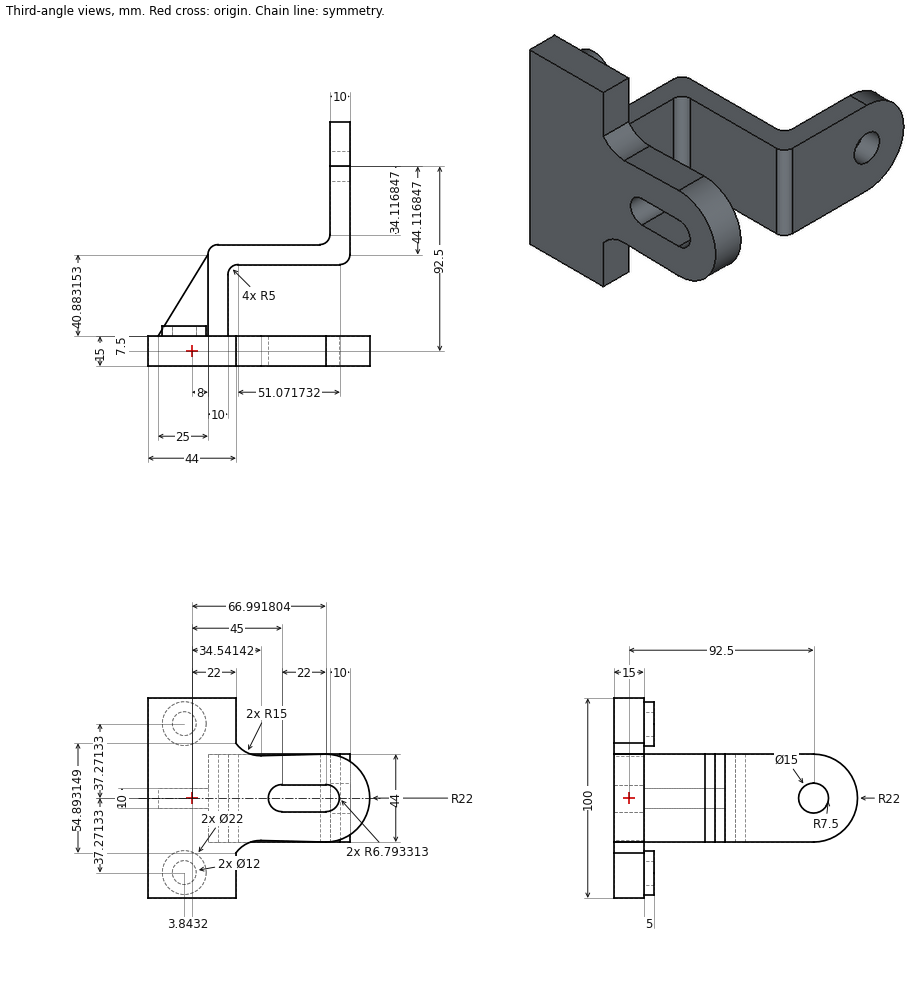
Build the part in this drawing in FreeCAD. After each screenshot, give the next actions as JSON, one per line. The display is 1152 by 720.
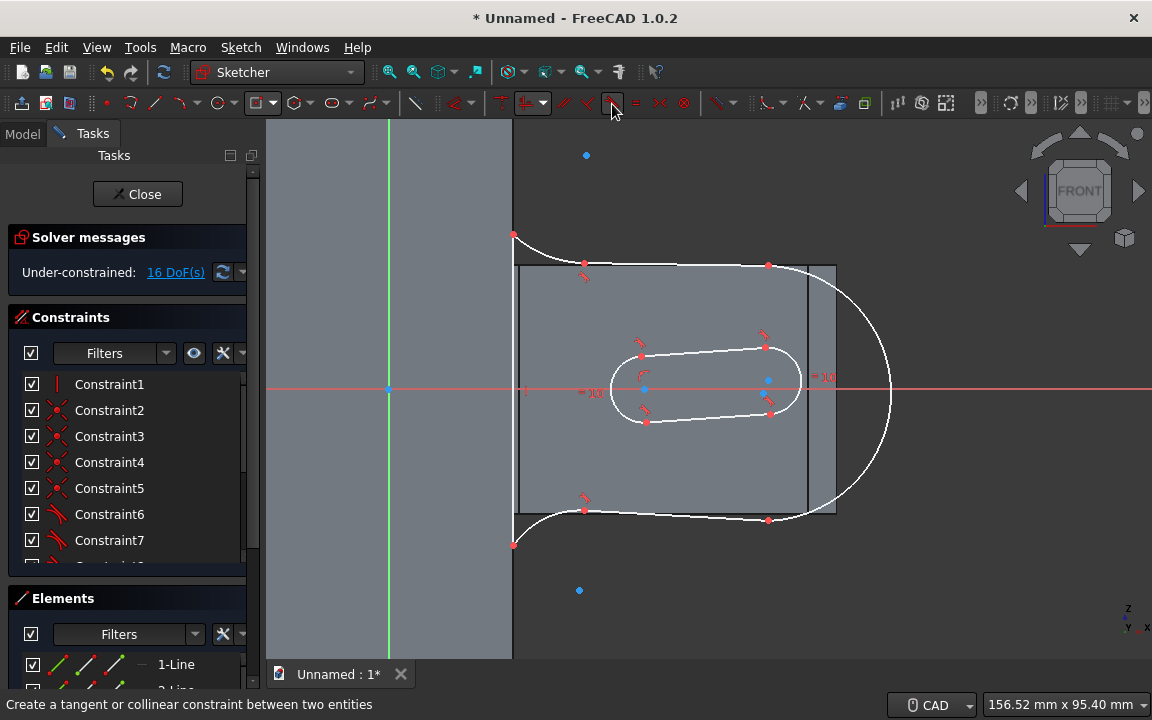
{"action": "left_click", "coordinate": [679, 354]}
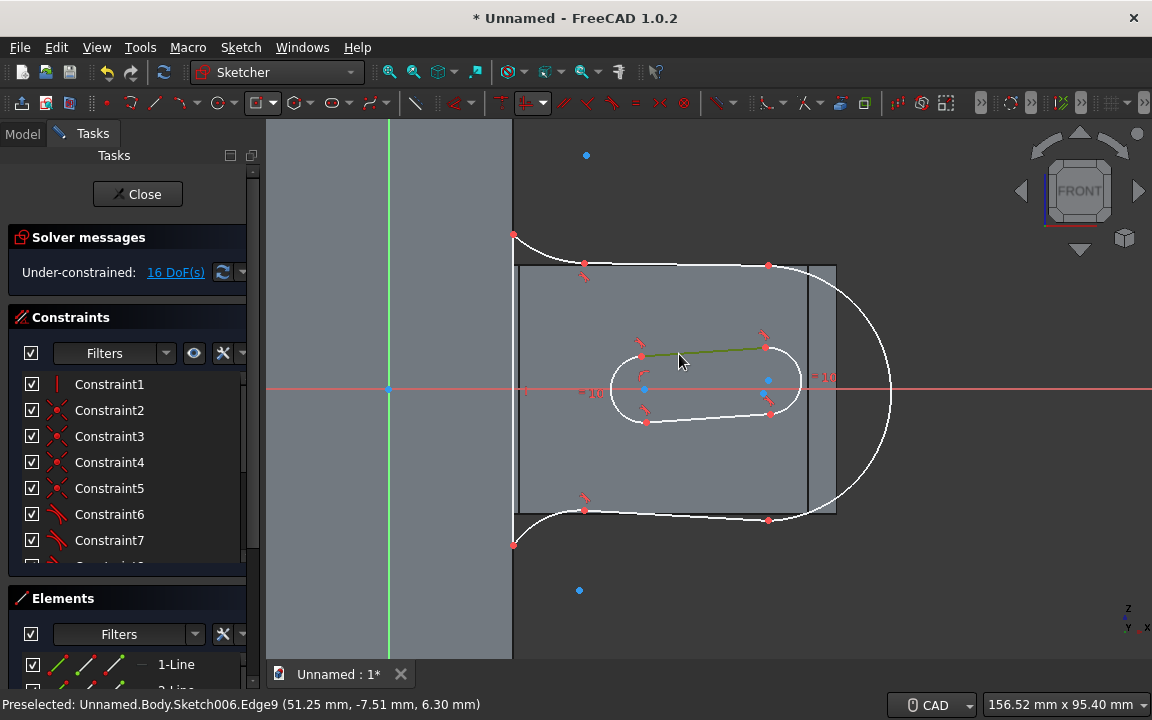
{"action": "key", "text": "h"}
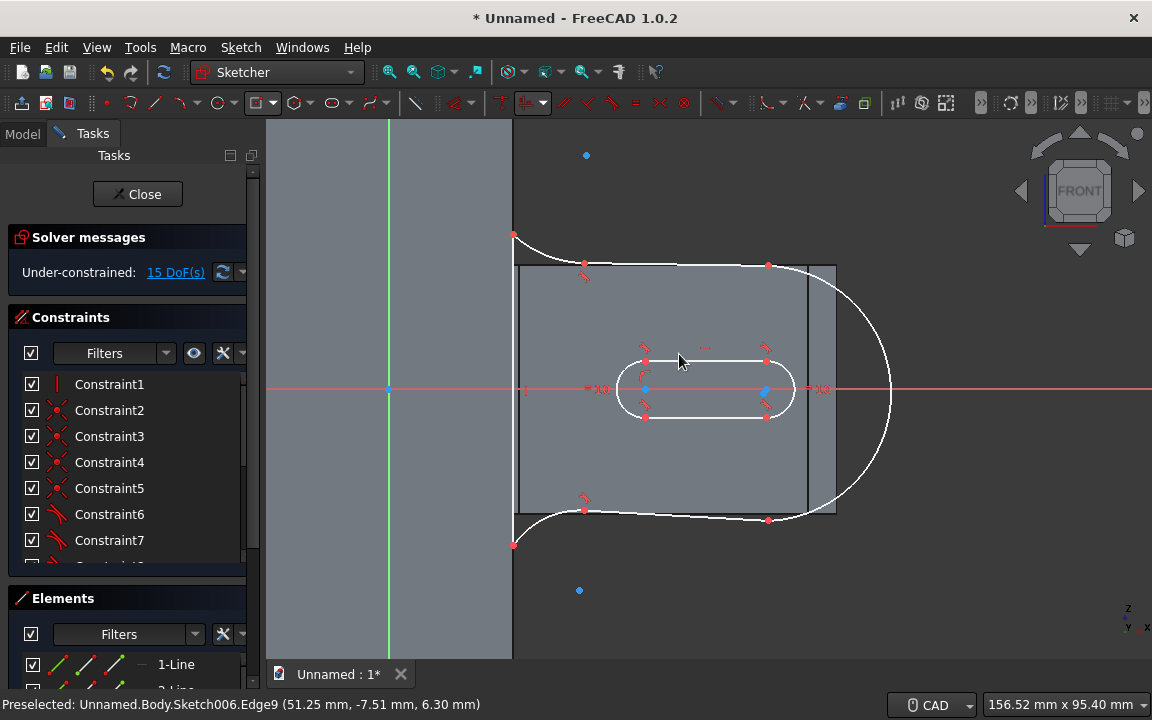
{"action": "left_click", "coordinate": [868, 467]}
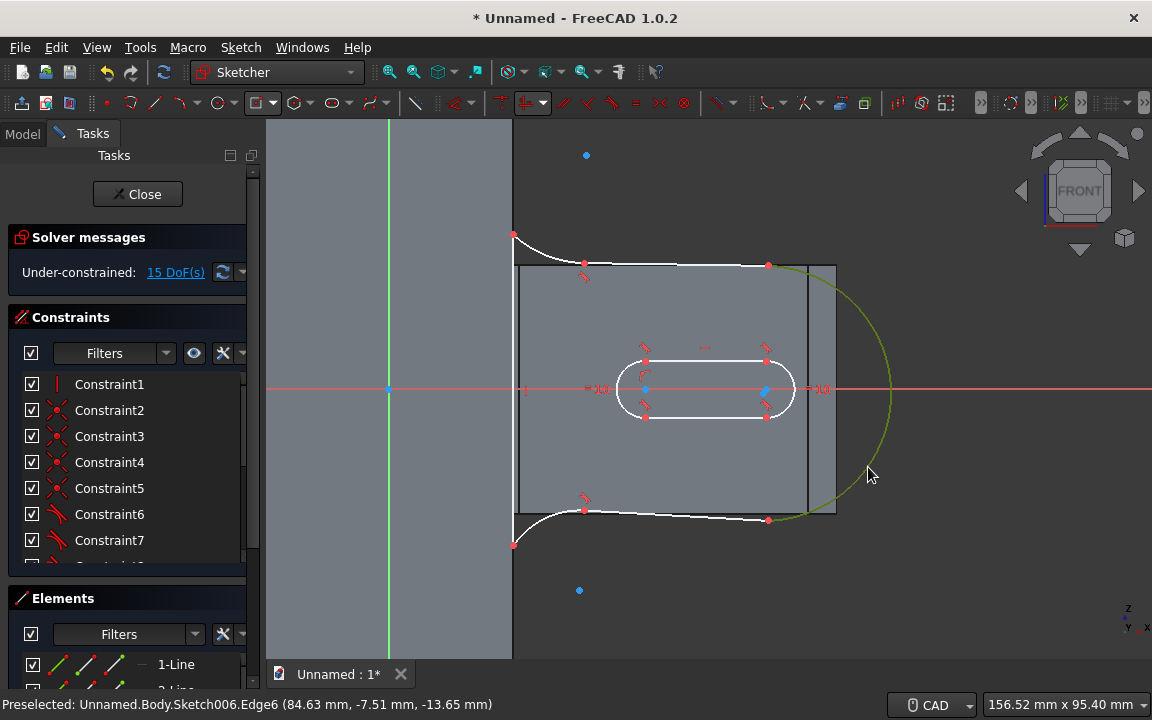
{"action": "left_click", "coordinate": [789, 406]}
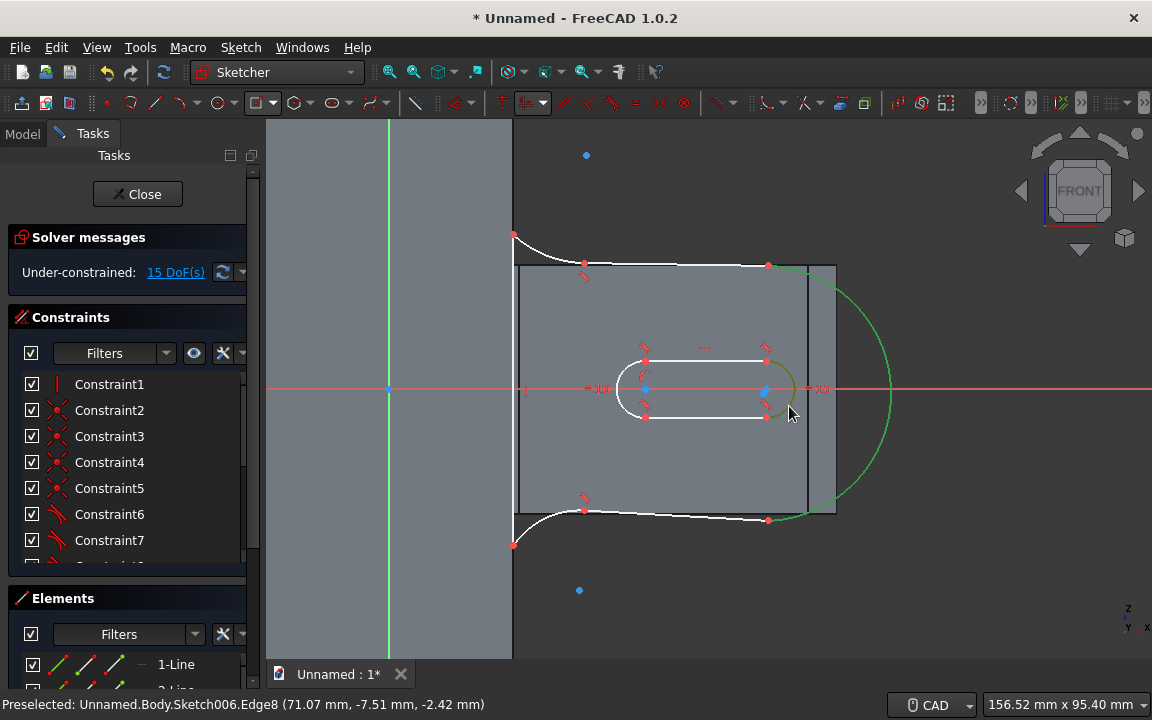
{"action": "left_click", "coordinate": [502, 104]}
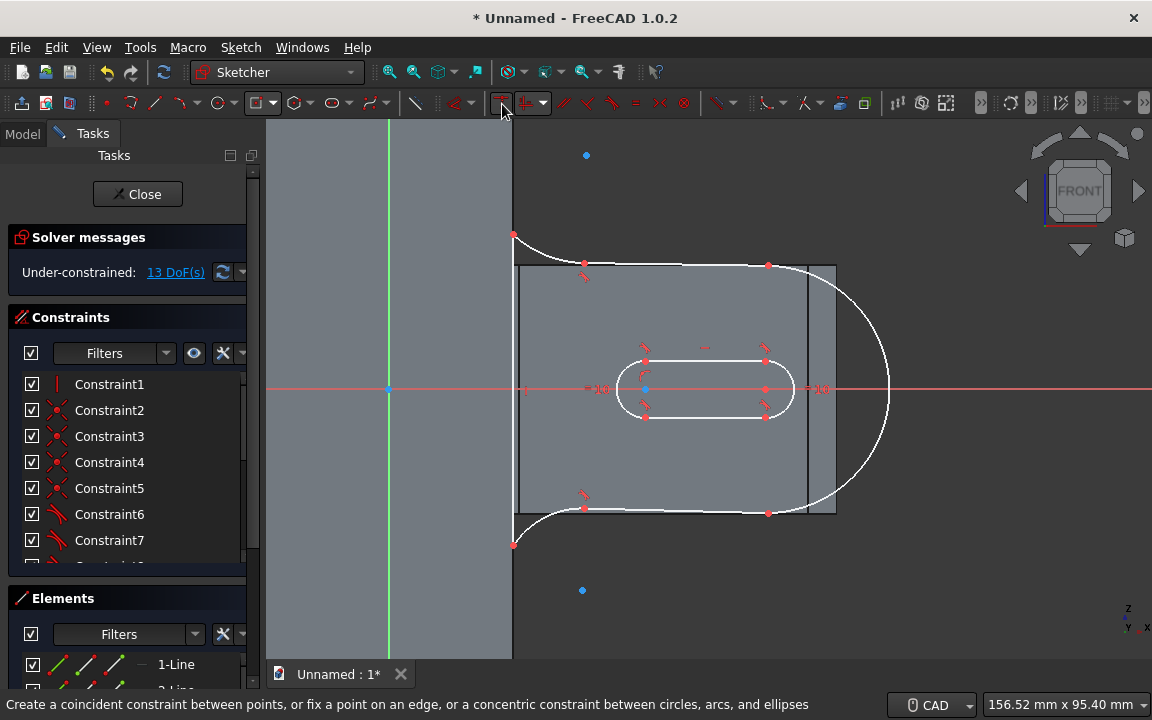
{"action": "left_click", "coordinate": [532, 249]}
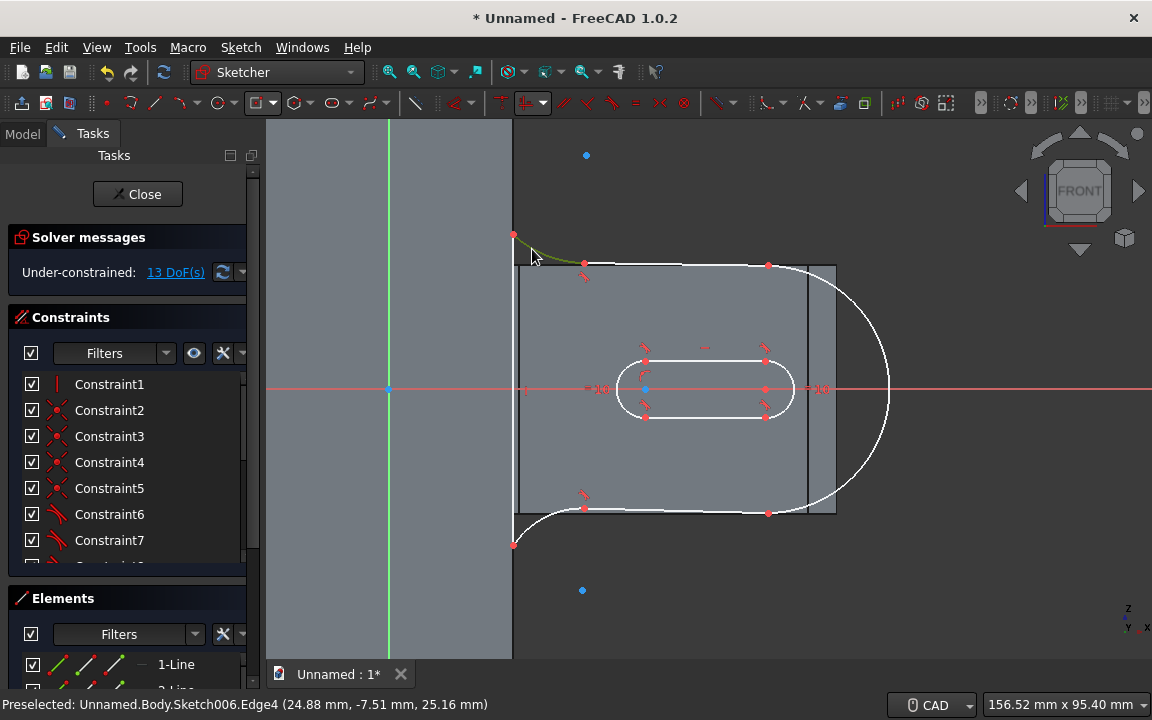
{"action": "left_click", "coordinate": [560, 512]}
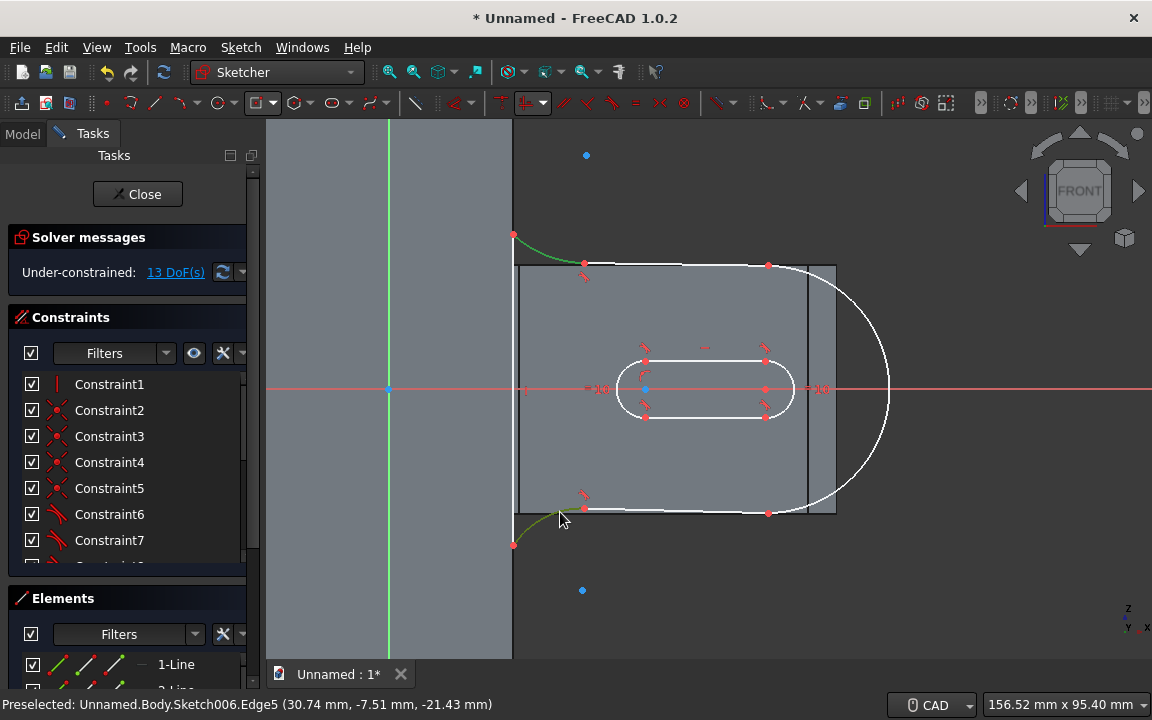
{"action": "left_click", "coordinate": [636, 104]}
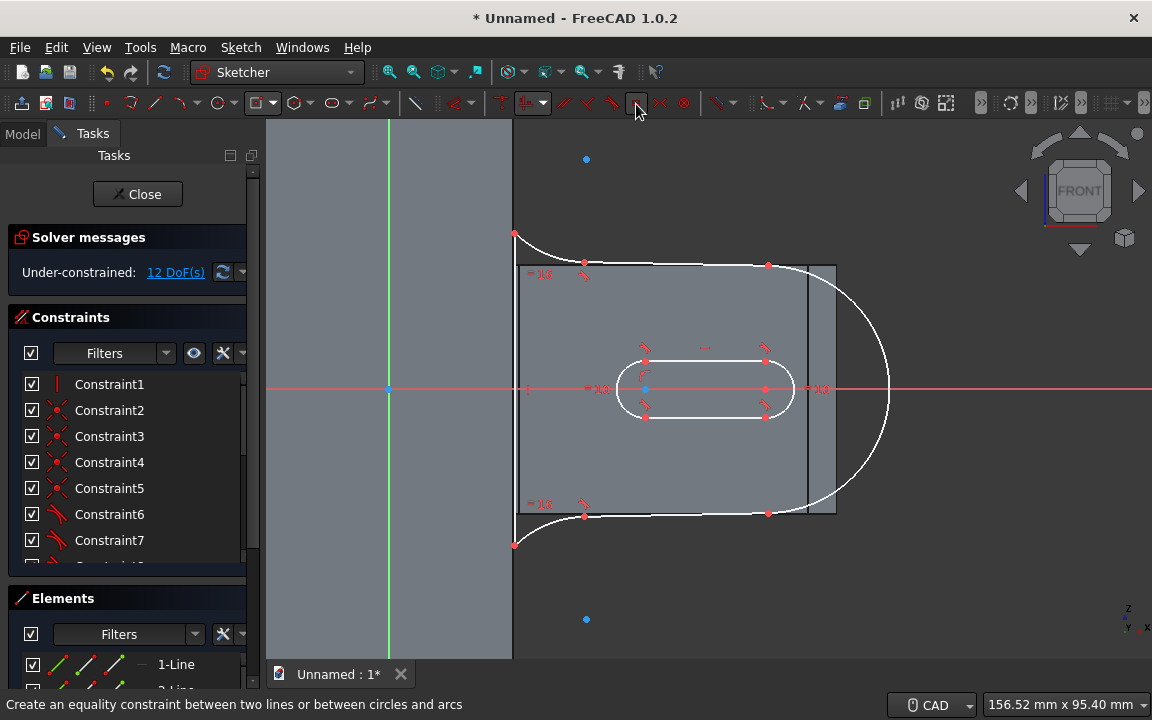
{"action": "left_click", "coordinate": [587, 160]}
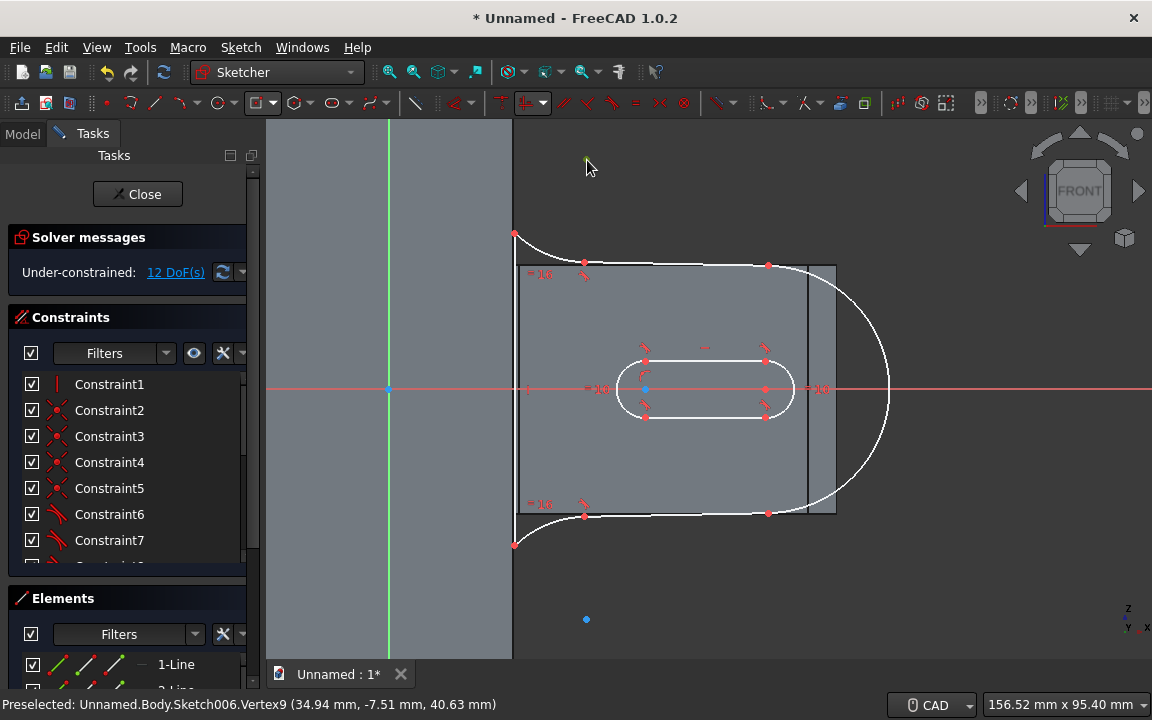
{"action": "left_click", "coordinate": [586, 619]}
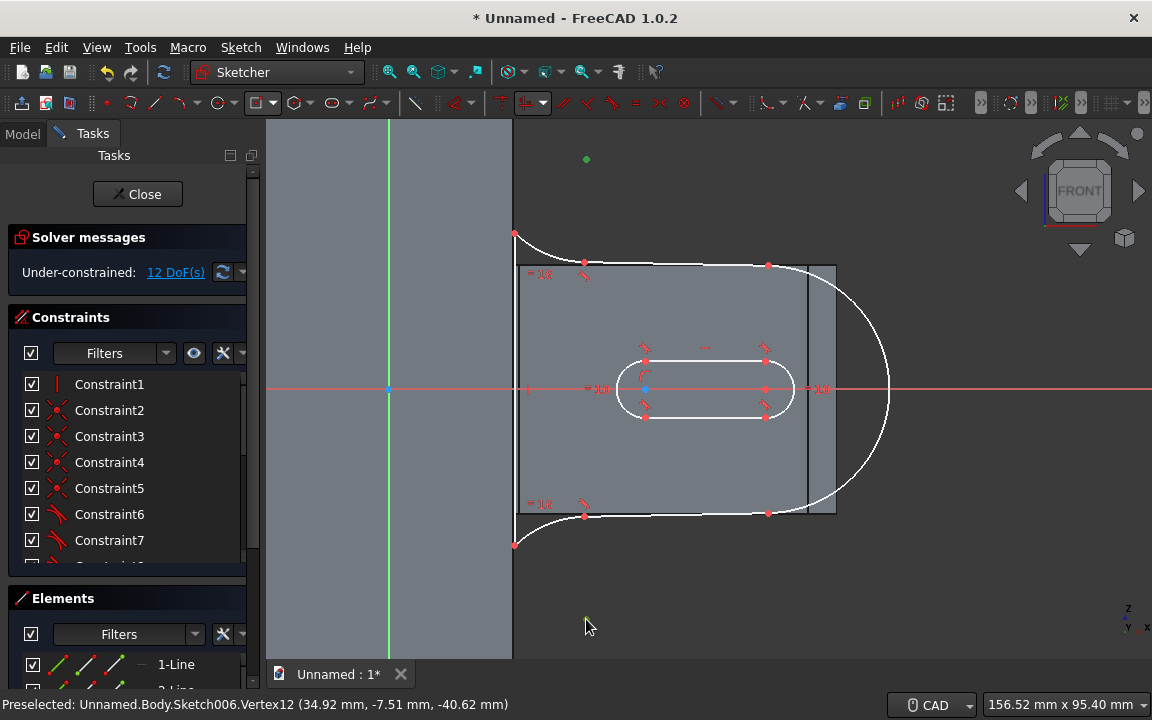
{"action": "left_click", "coordinate": [344, 389]}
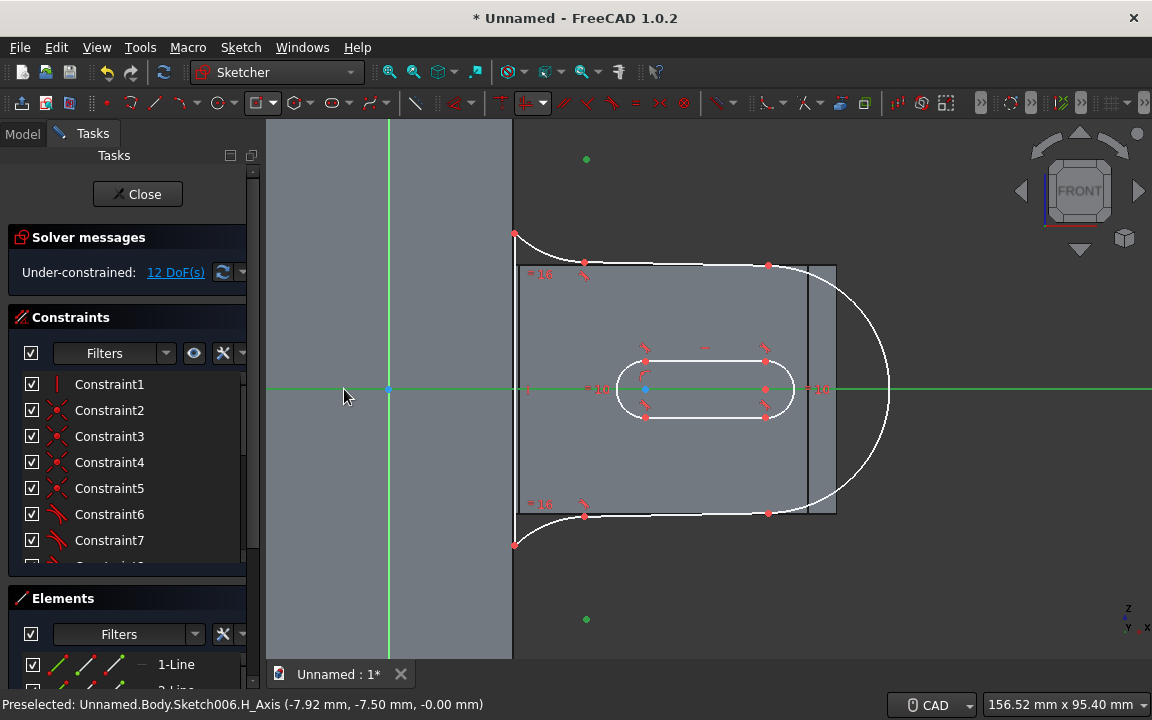
{"action": "left_click", "coordinate": [660, 104]}